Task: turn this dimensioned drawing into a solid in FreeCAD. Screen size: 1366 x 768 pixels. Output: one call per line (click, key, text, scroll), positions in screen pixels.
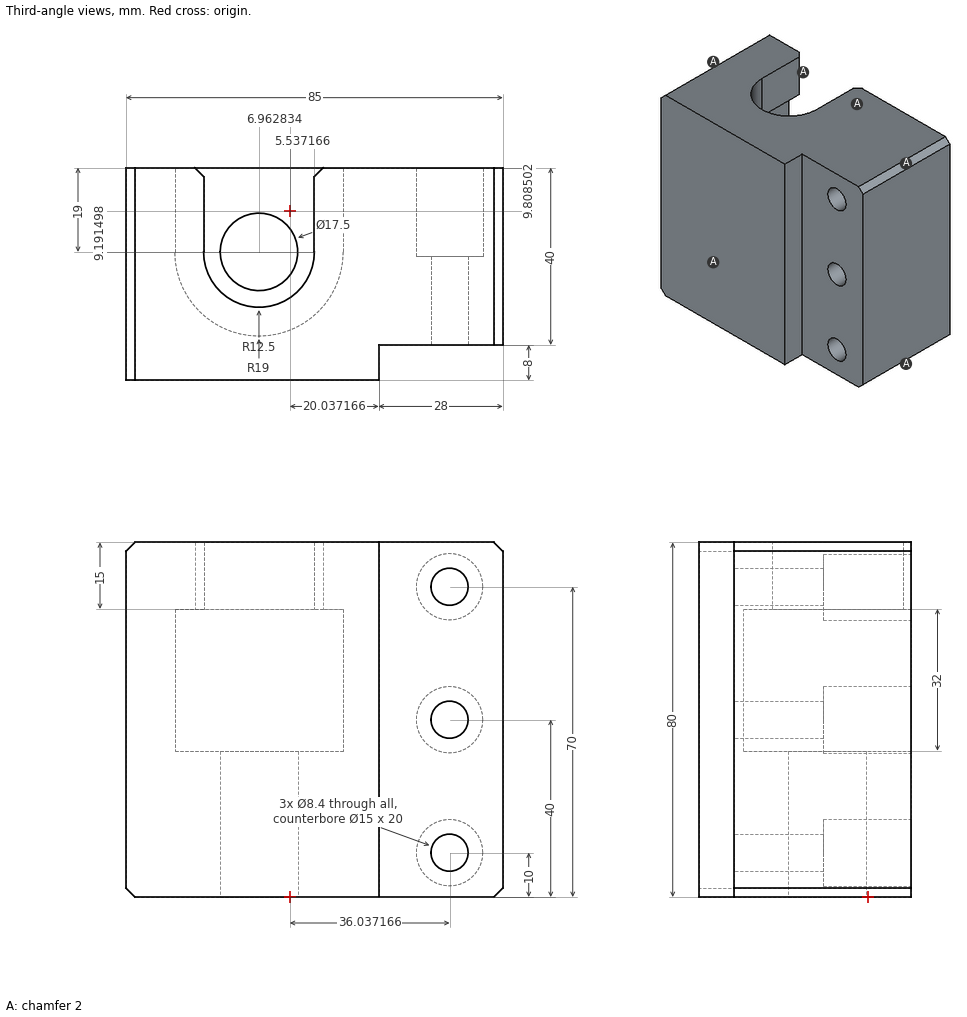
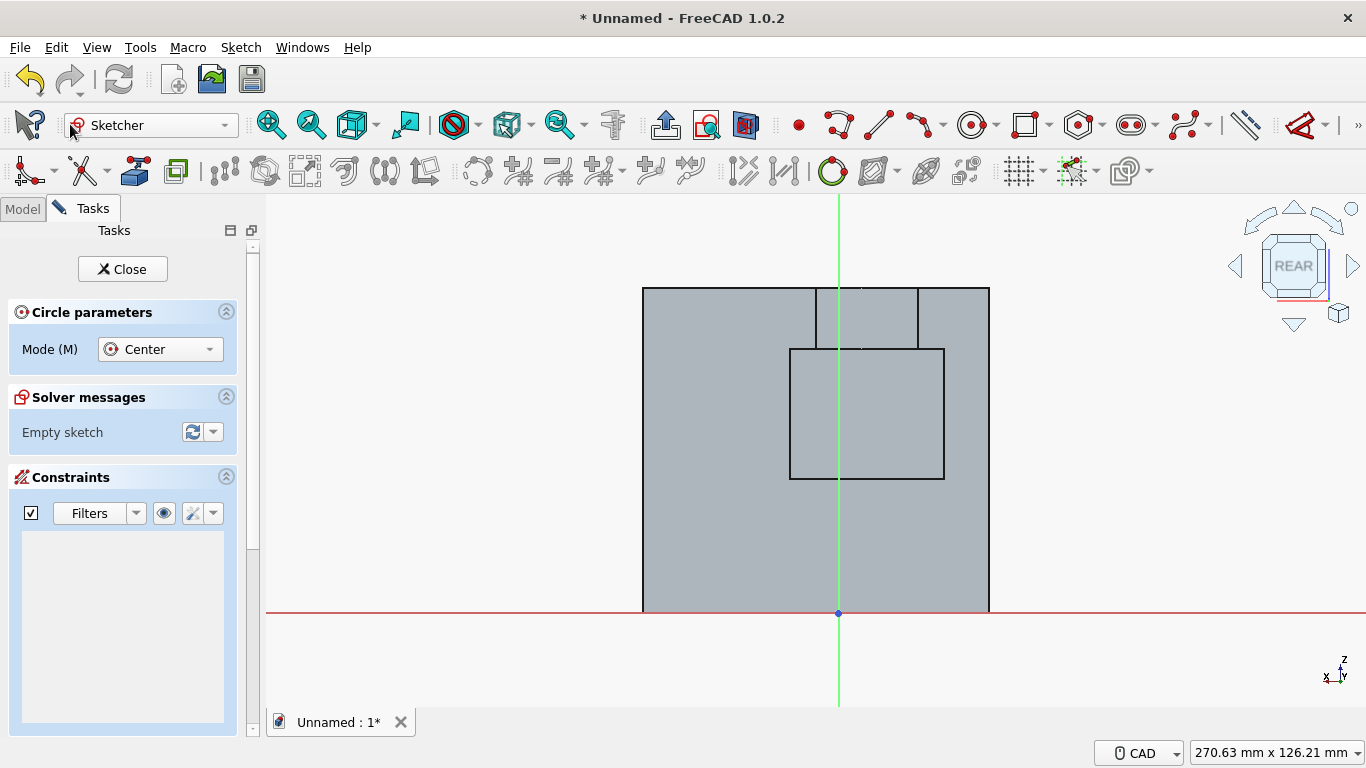
scroll(692, 572, up, 2)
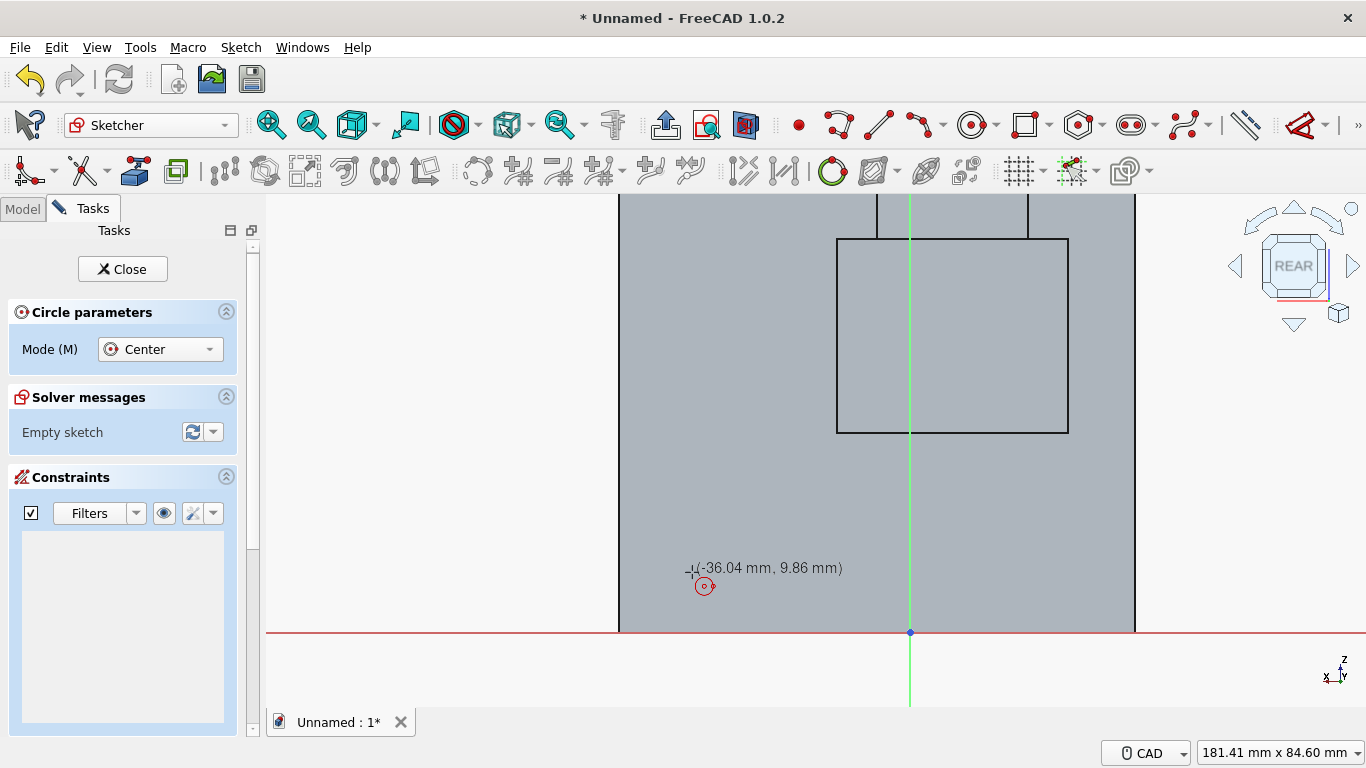
click(692, 572)
move(710, 554)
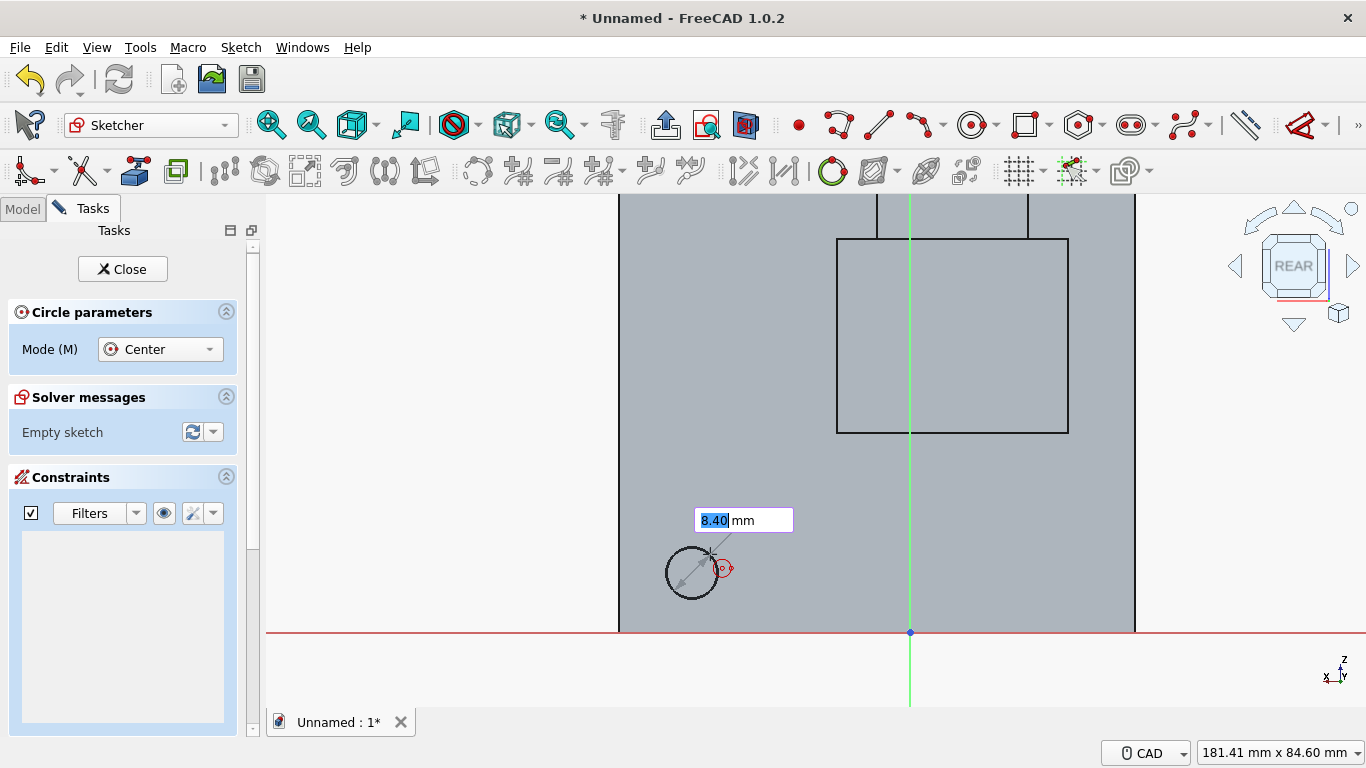
text(8.4)
key(Return)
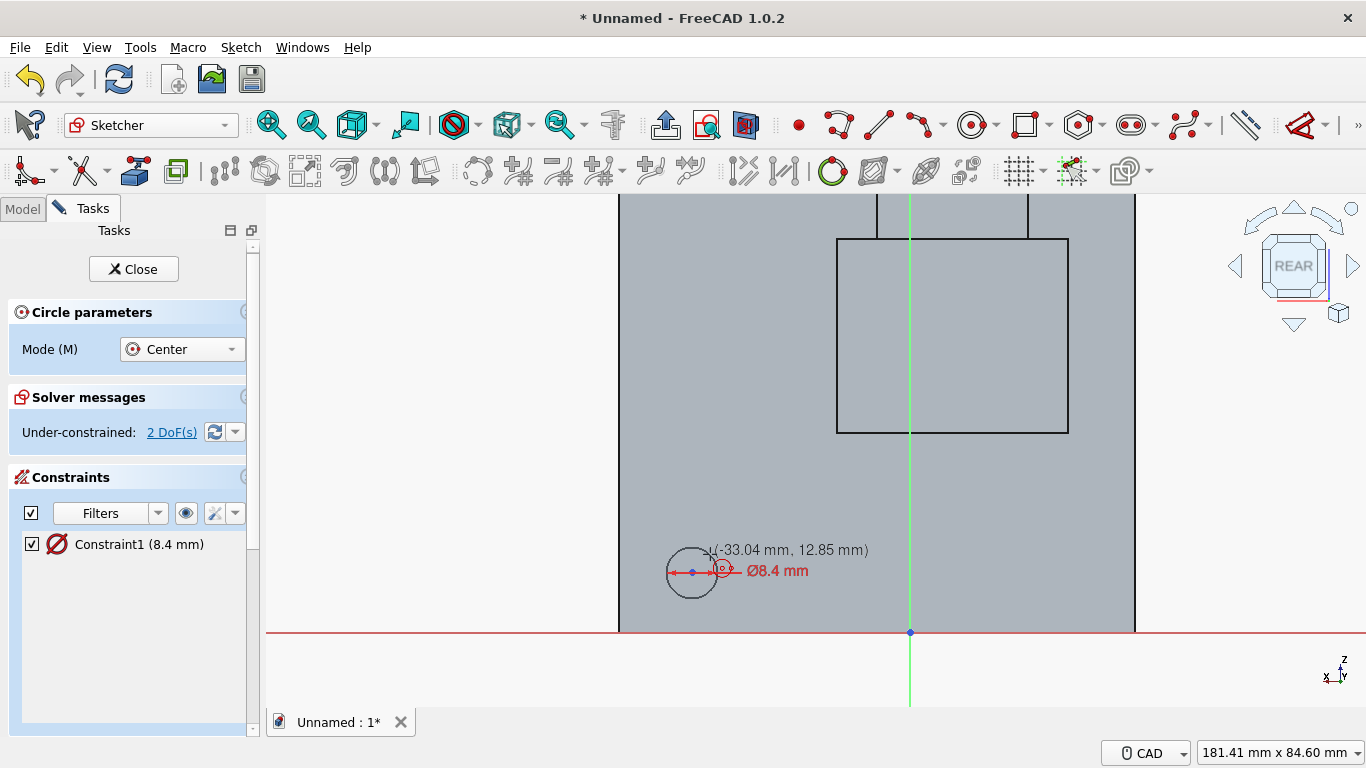
click(692, 390)
move(710, 372)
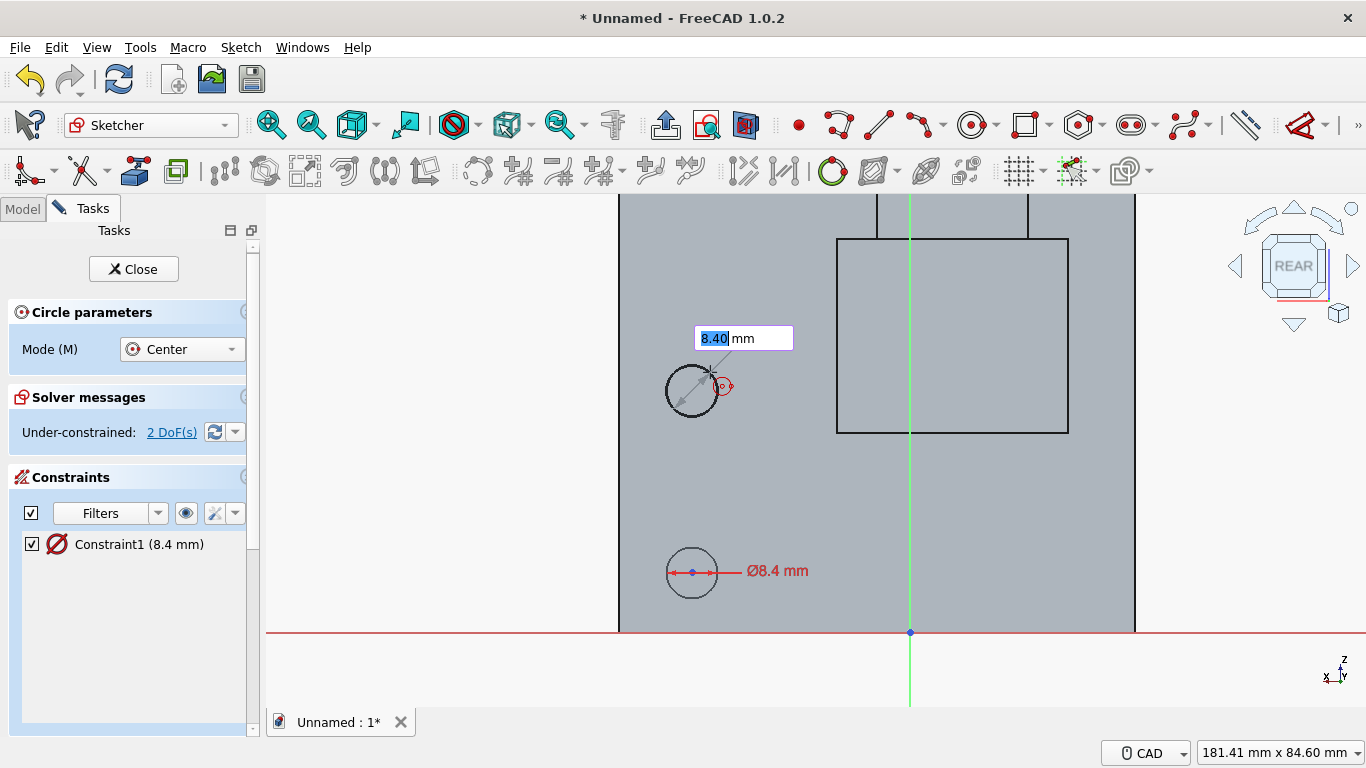
text(8.4)
key(Return)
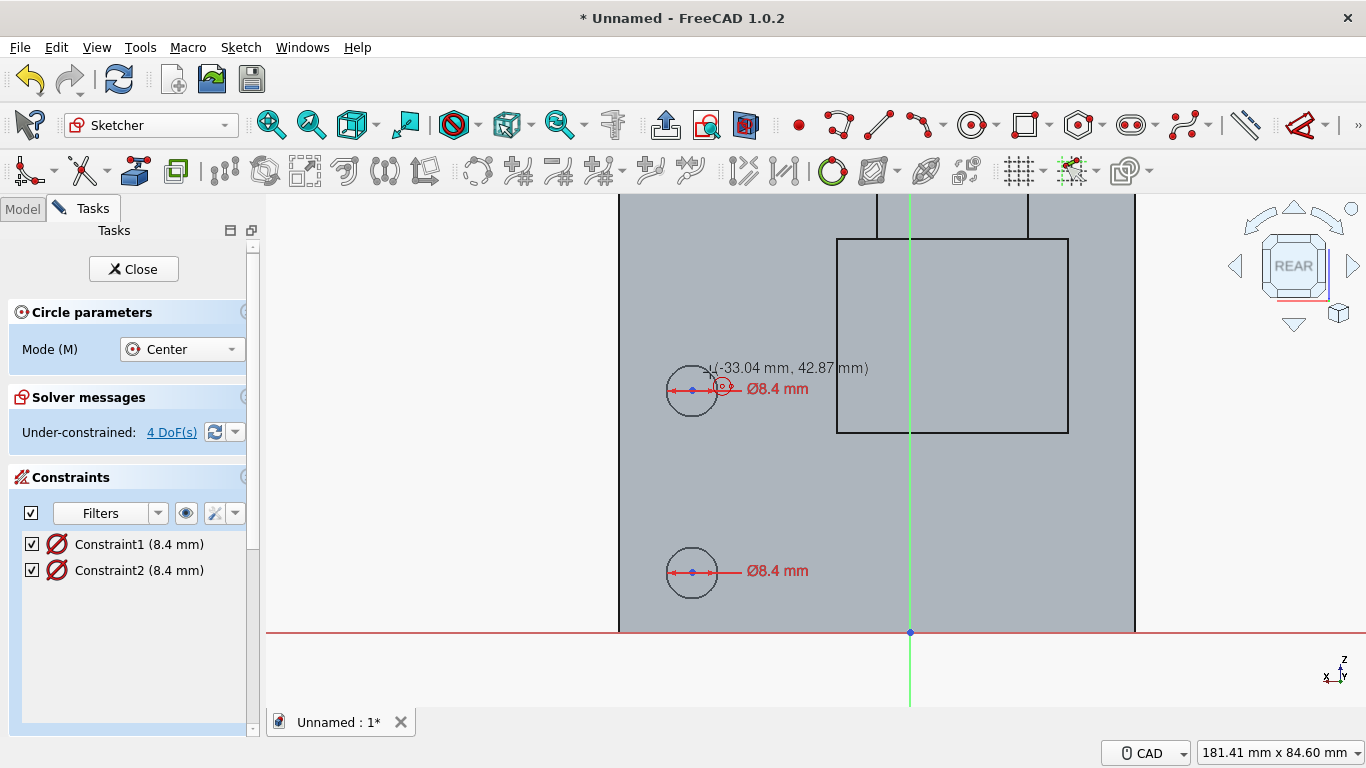
scroll(664, 537, down, 2)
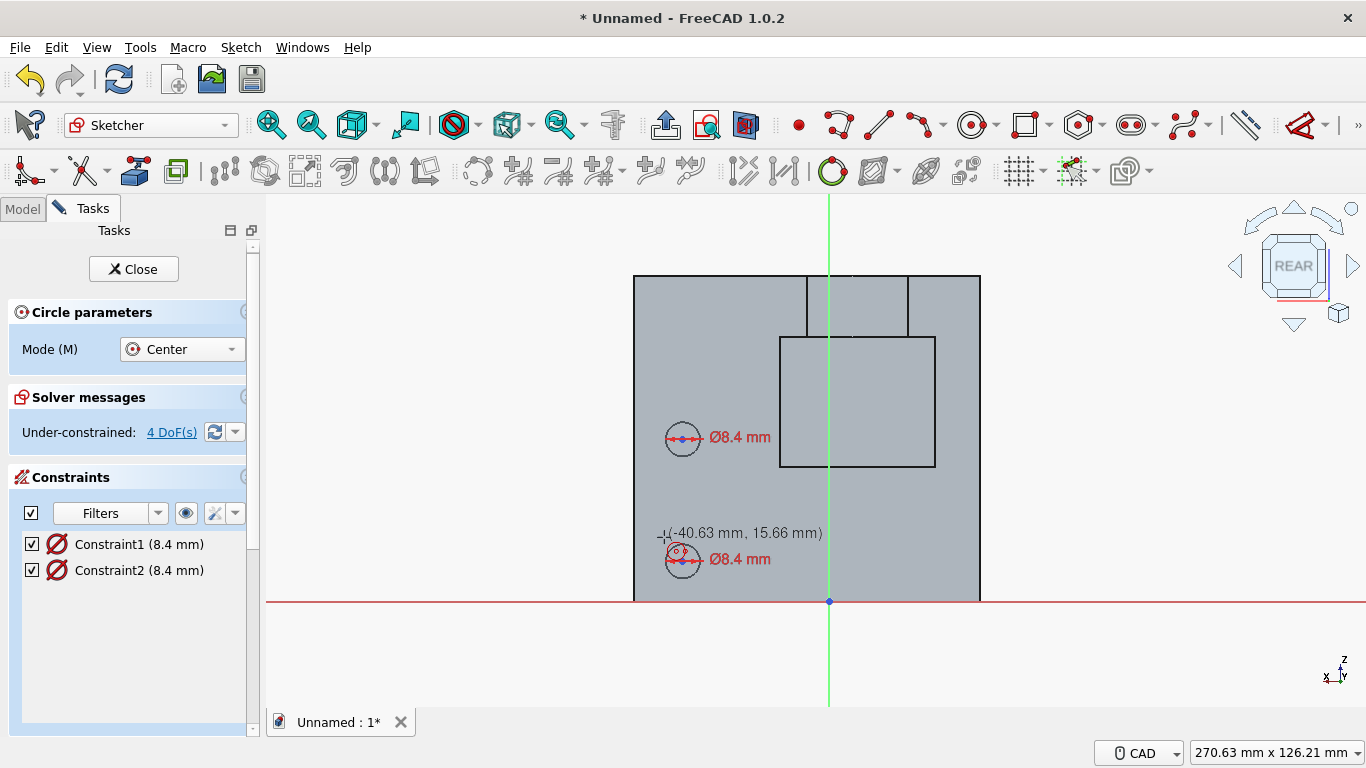
scroll(683, 317, up, 2)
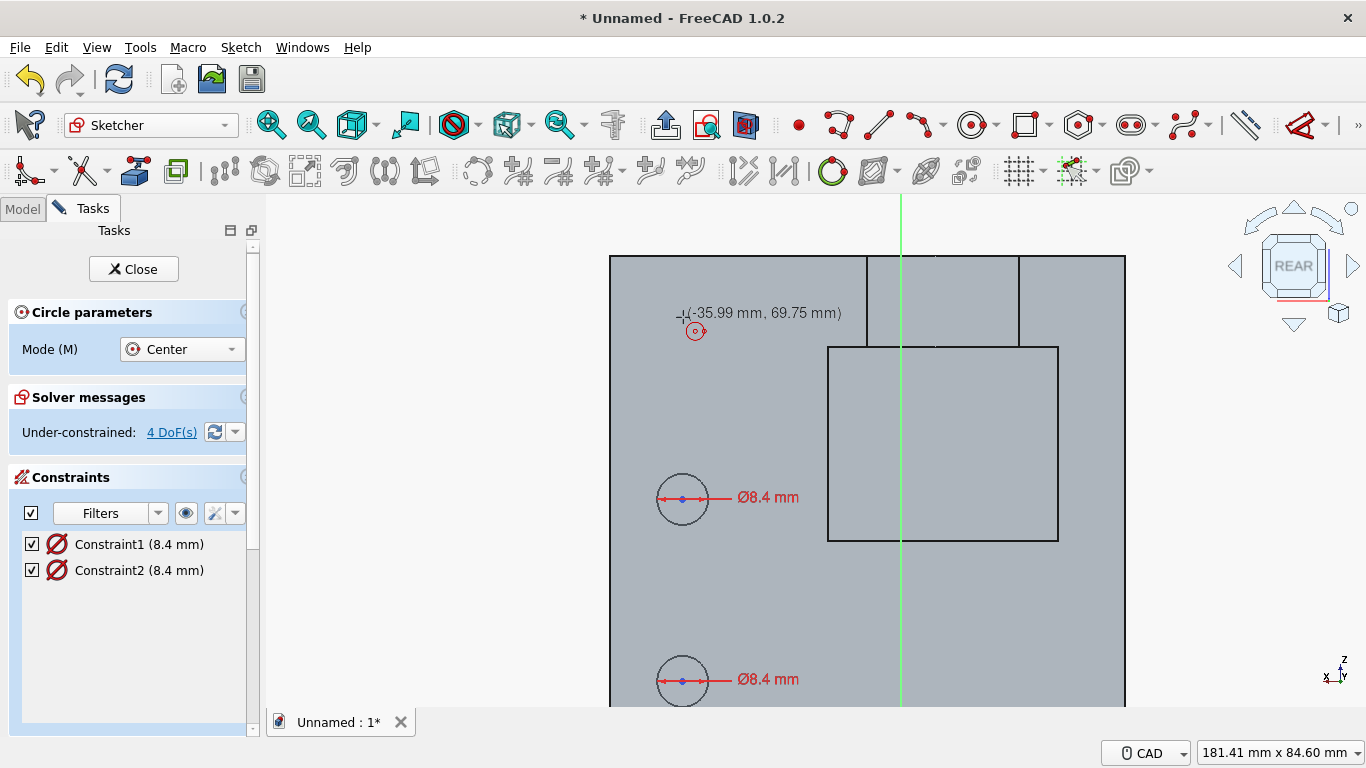
click(682, 317)
move(701, 299)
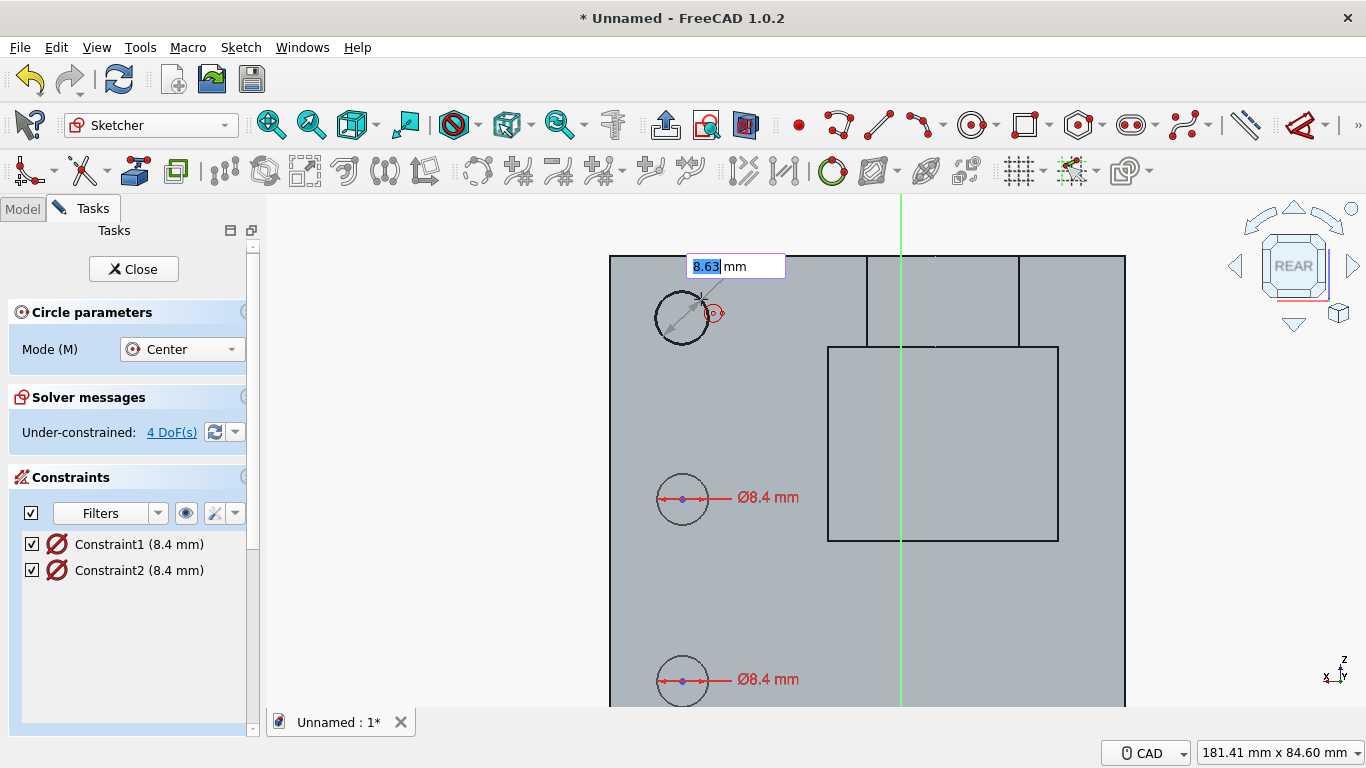
text(8.4)
key(Return)
key(Escape)